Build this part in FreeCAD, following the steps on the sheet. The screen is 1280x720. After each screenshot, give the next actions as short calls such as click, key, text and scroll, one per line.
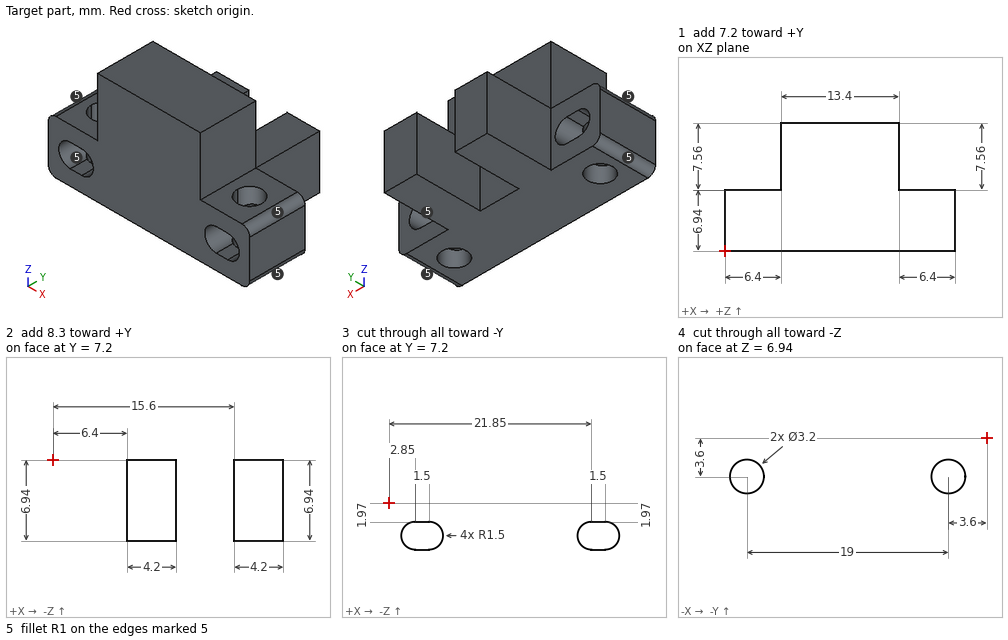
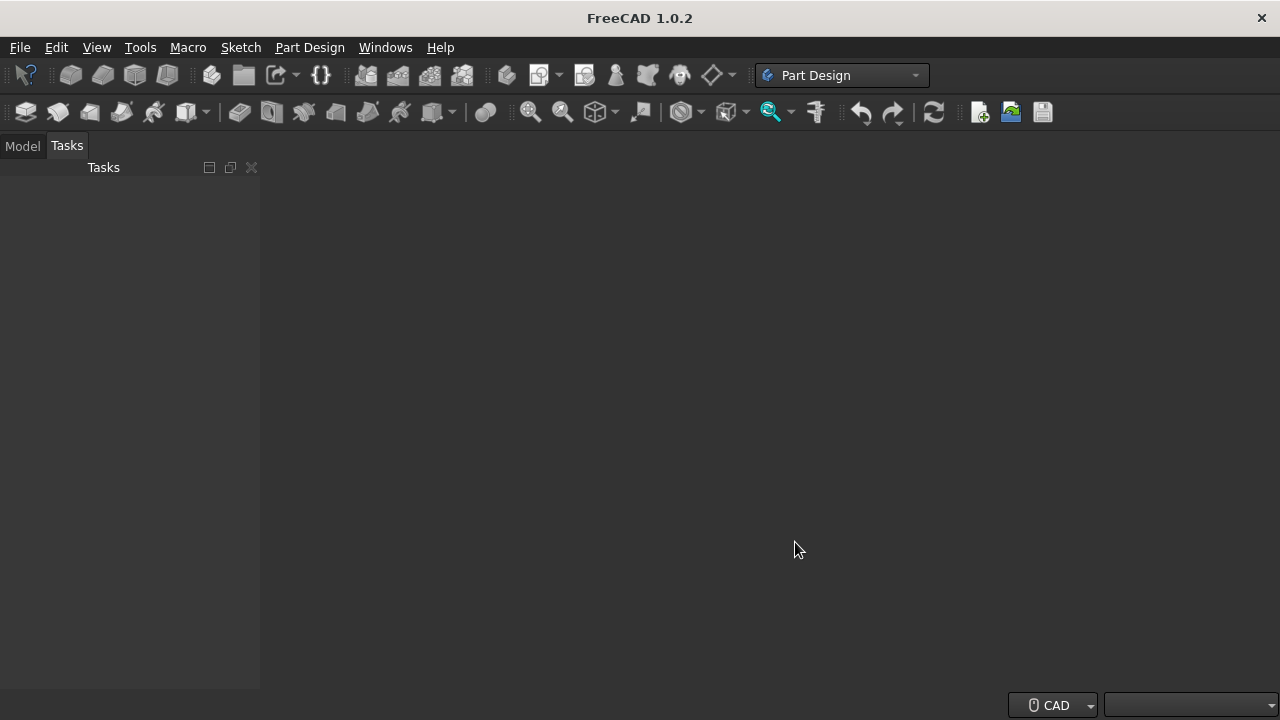
click(980, 112)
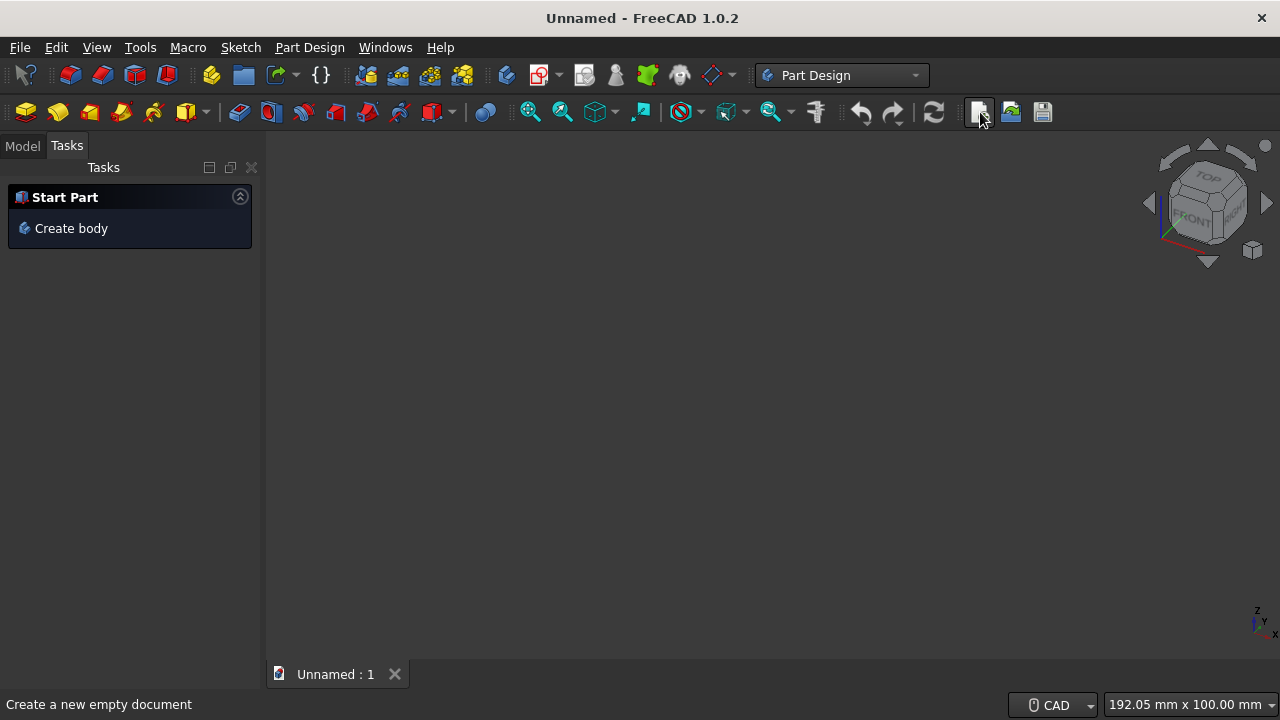
click(540, 76)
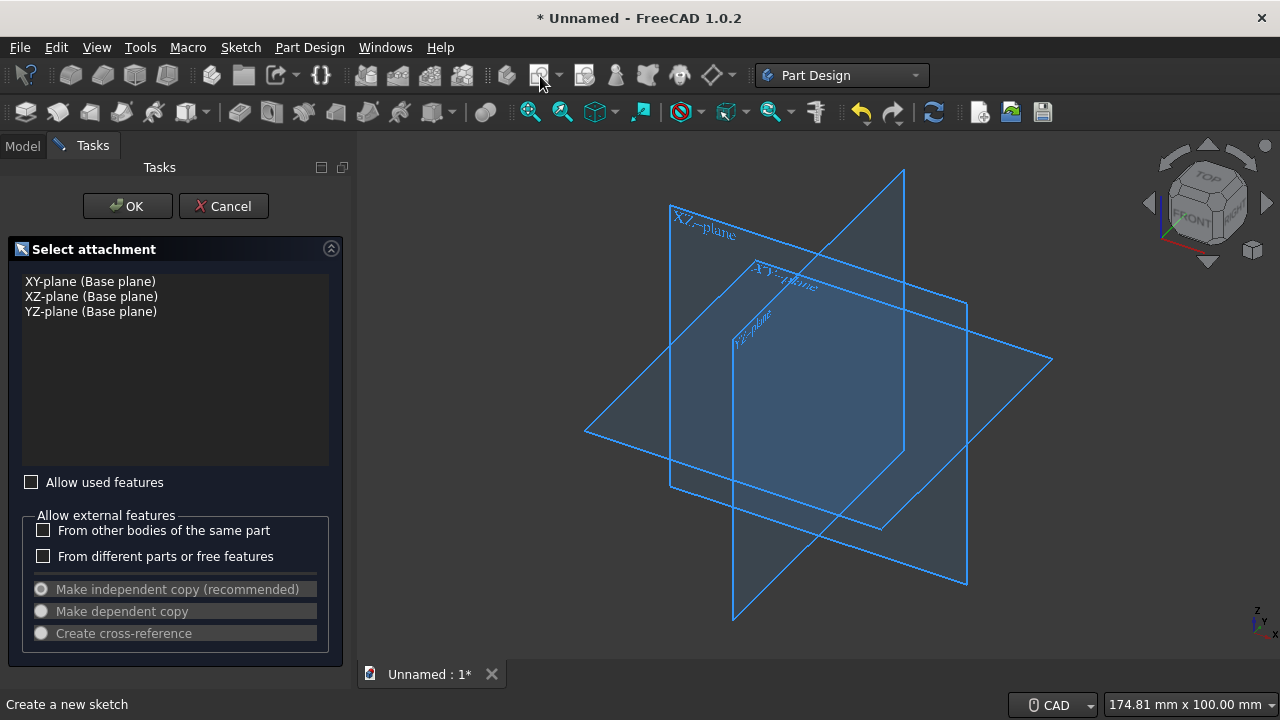
click(82, 296)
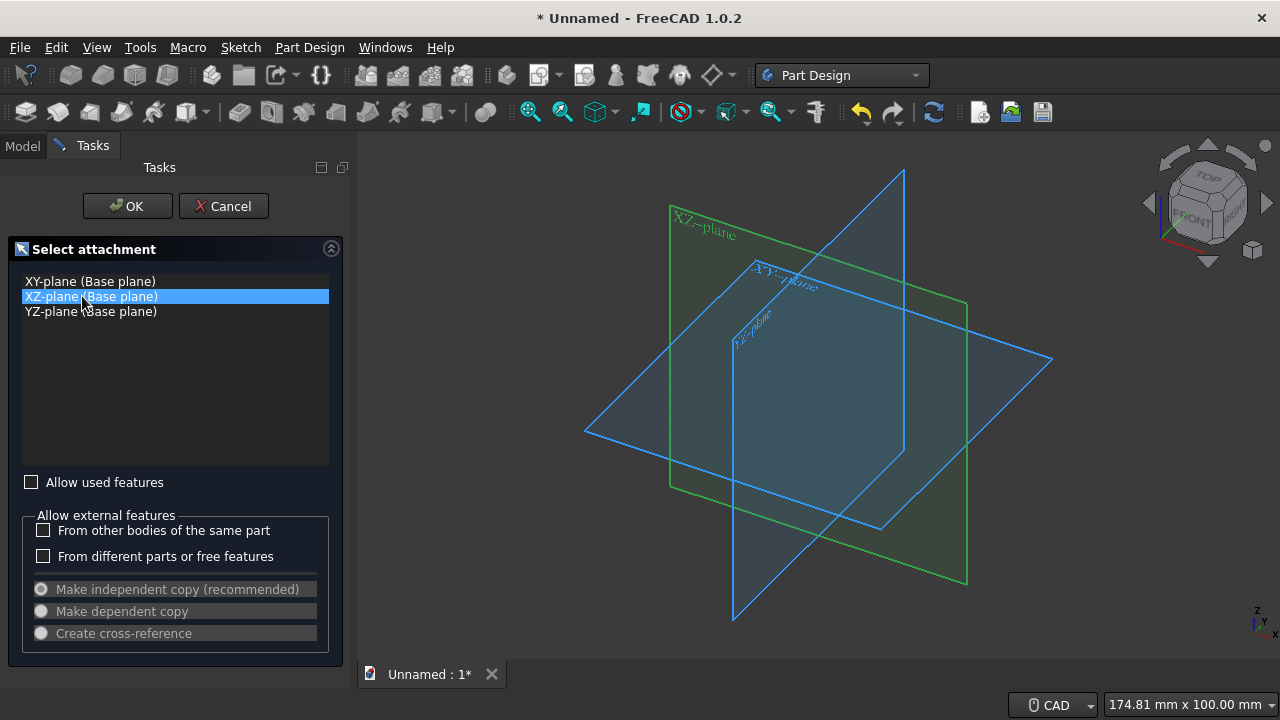
click(128, 206)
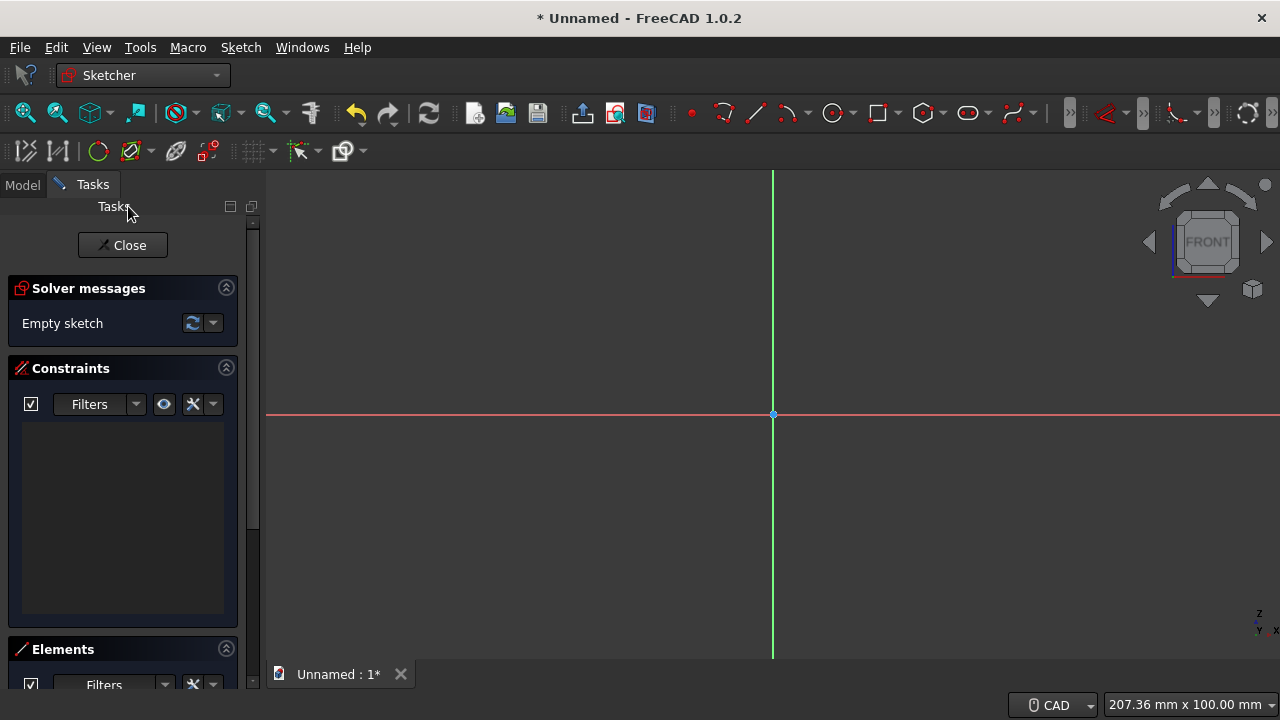
scroll(880, 367, up, 7)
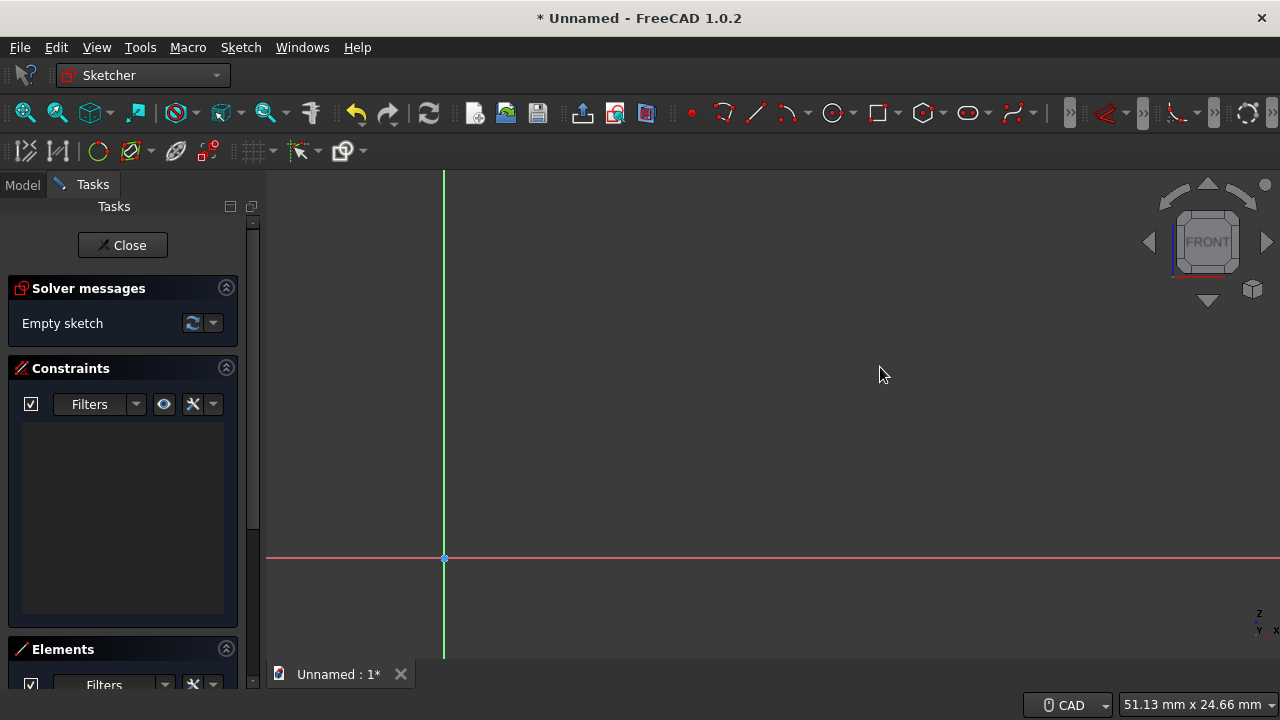
click(724, 114)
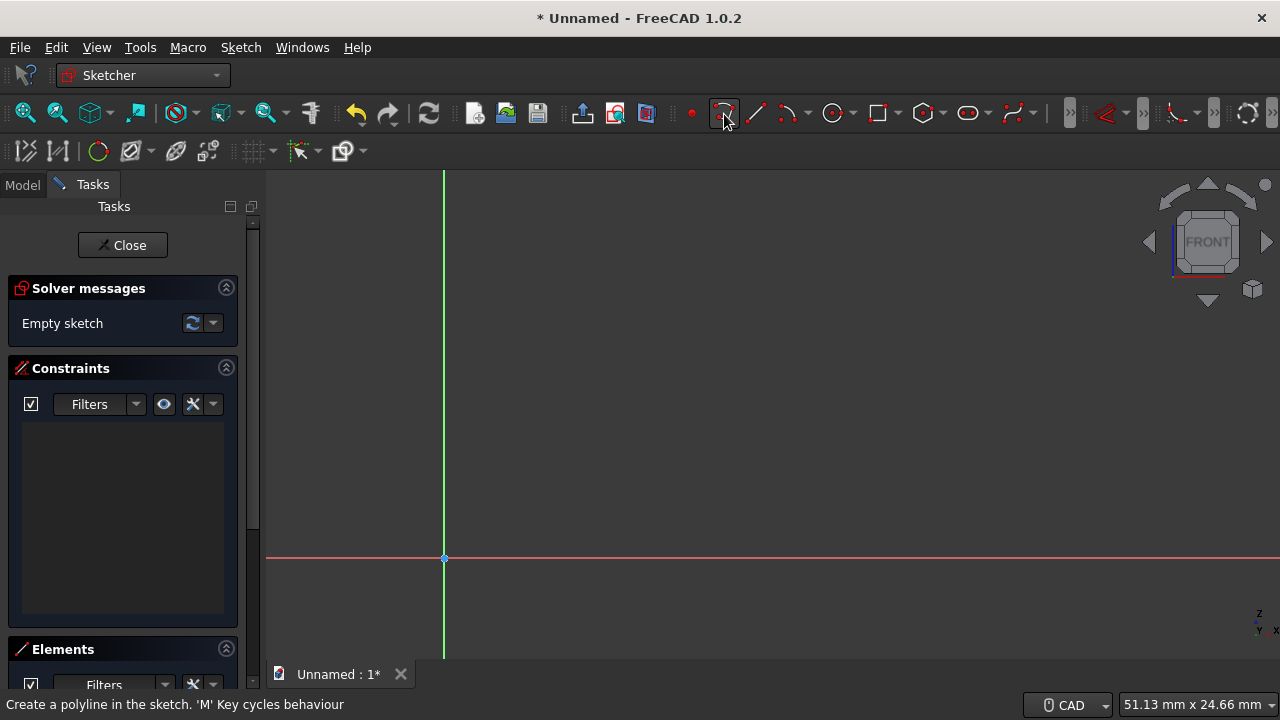
click(444, 558)
click(453, 421)
click(571, 421)
click(571, 271)
click(837, 271)
click(837, 421)
click(964, 421)
click(964, 549)
click(444, 558)
key(Escape)
key(Escape)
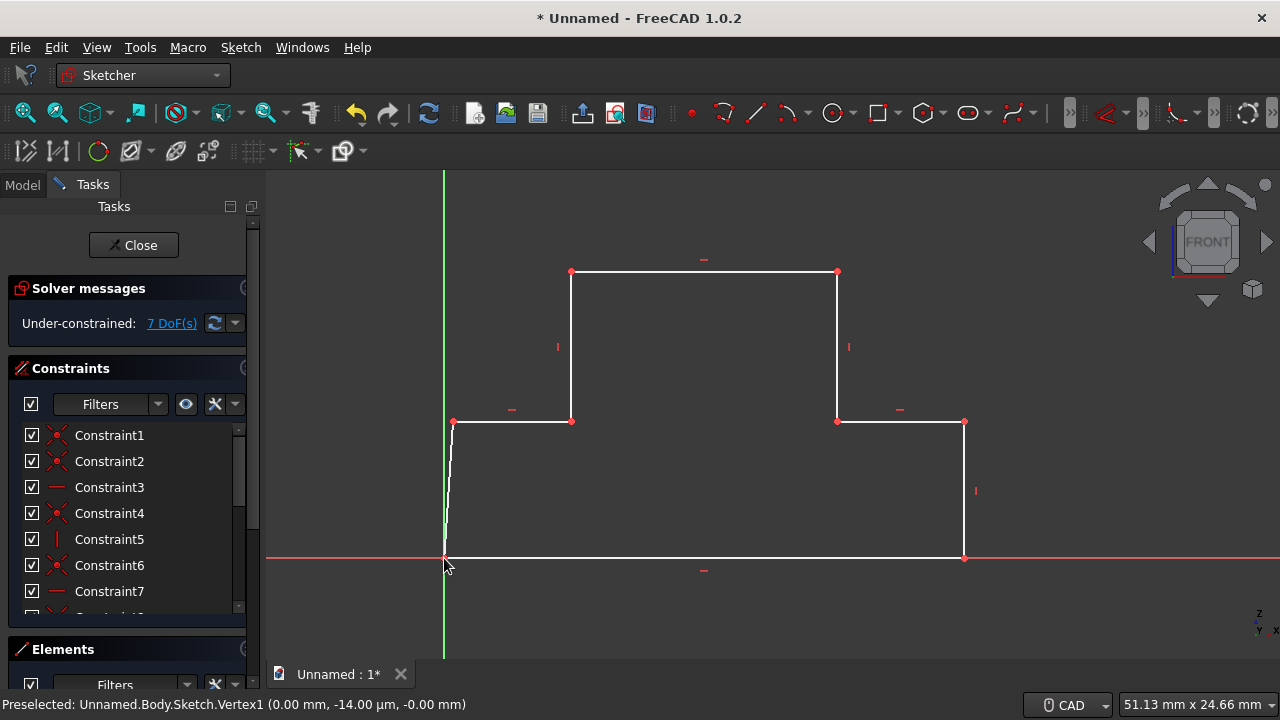
click(447, 517)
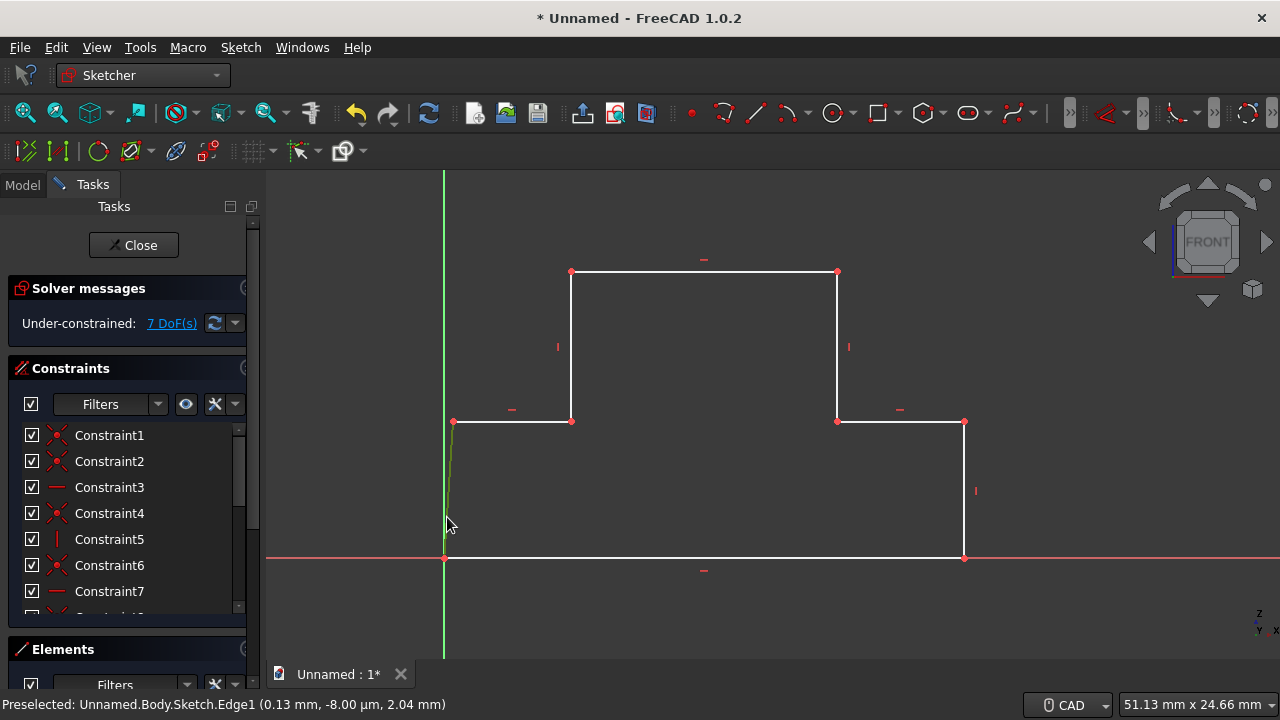
key(v)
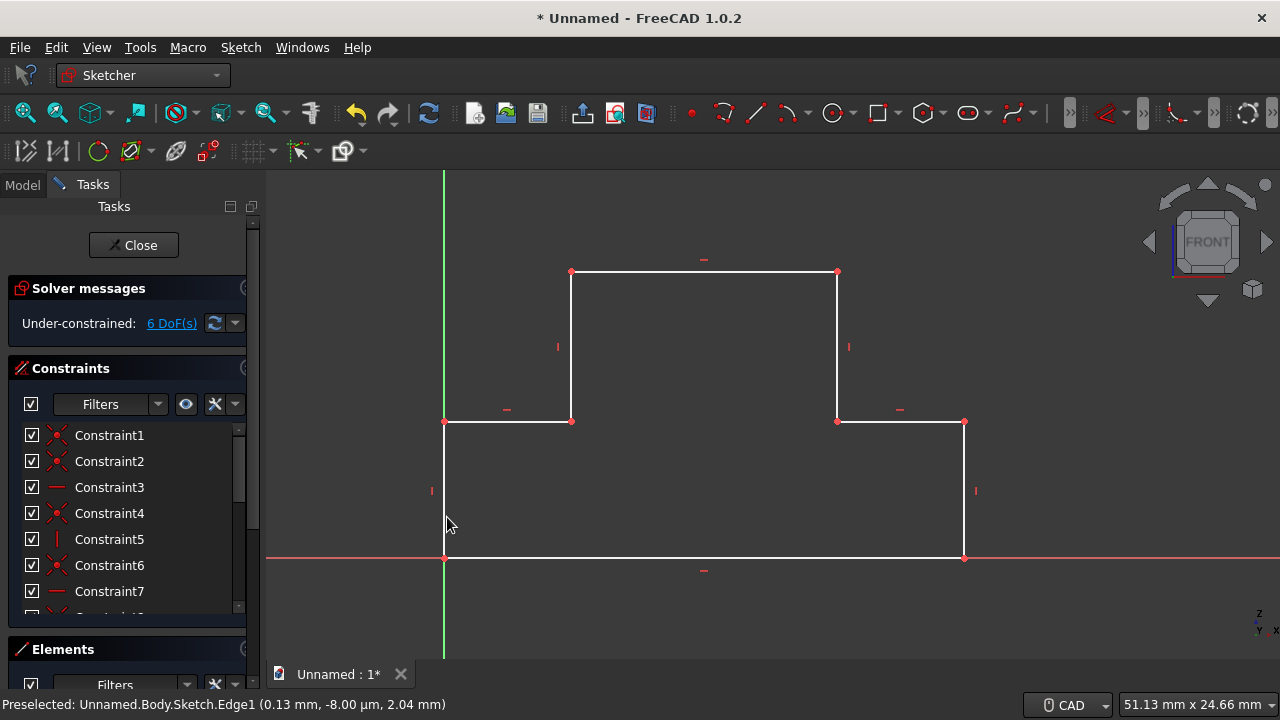
click(1106, 114)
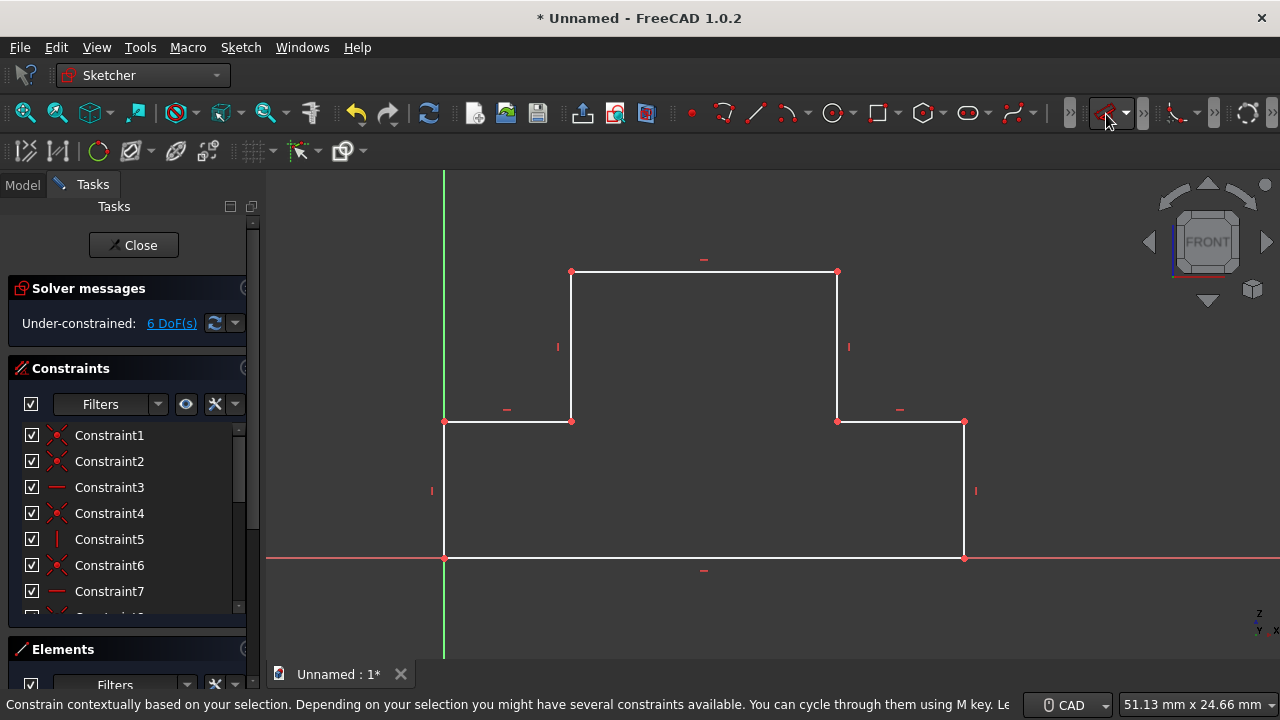
click(482, 422)
click(508, 456)